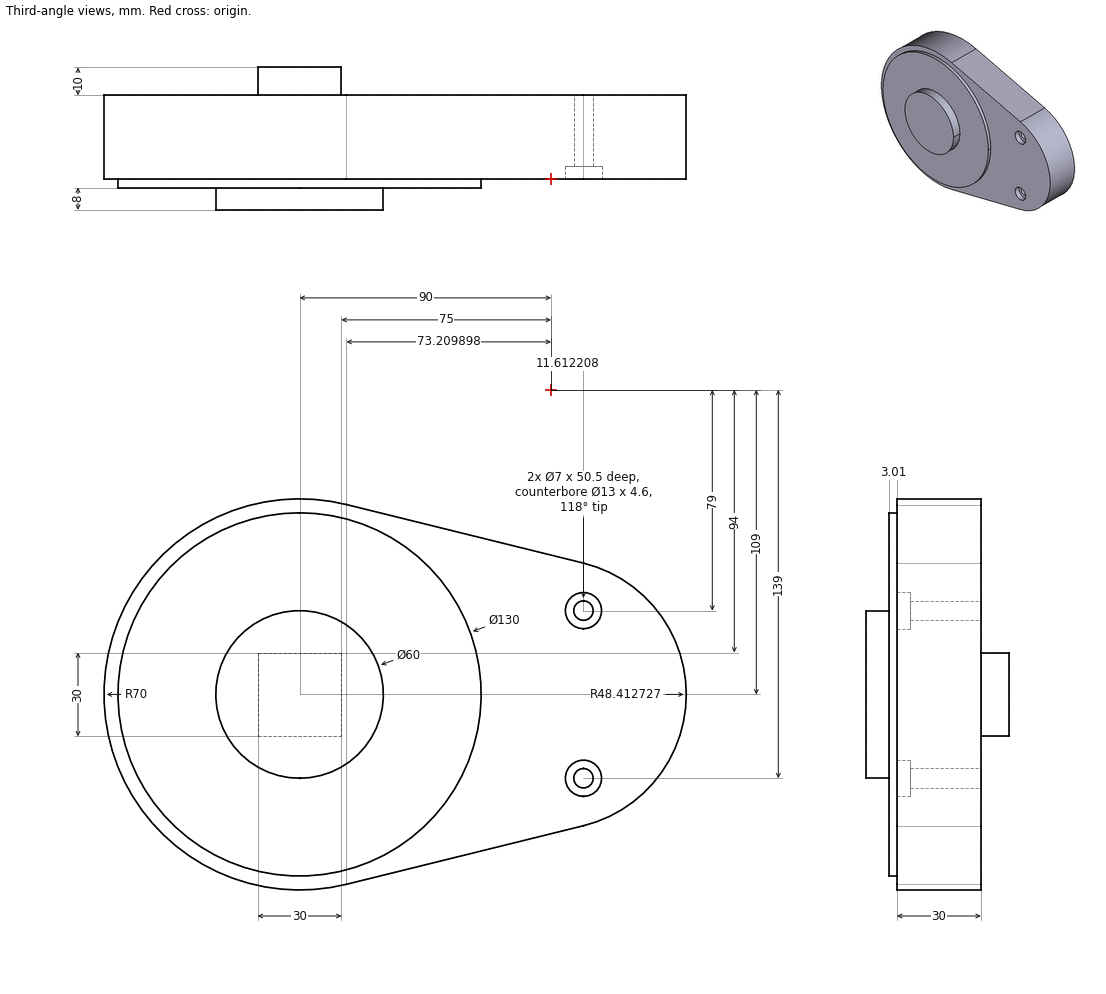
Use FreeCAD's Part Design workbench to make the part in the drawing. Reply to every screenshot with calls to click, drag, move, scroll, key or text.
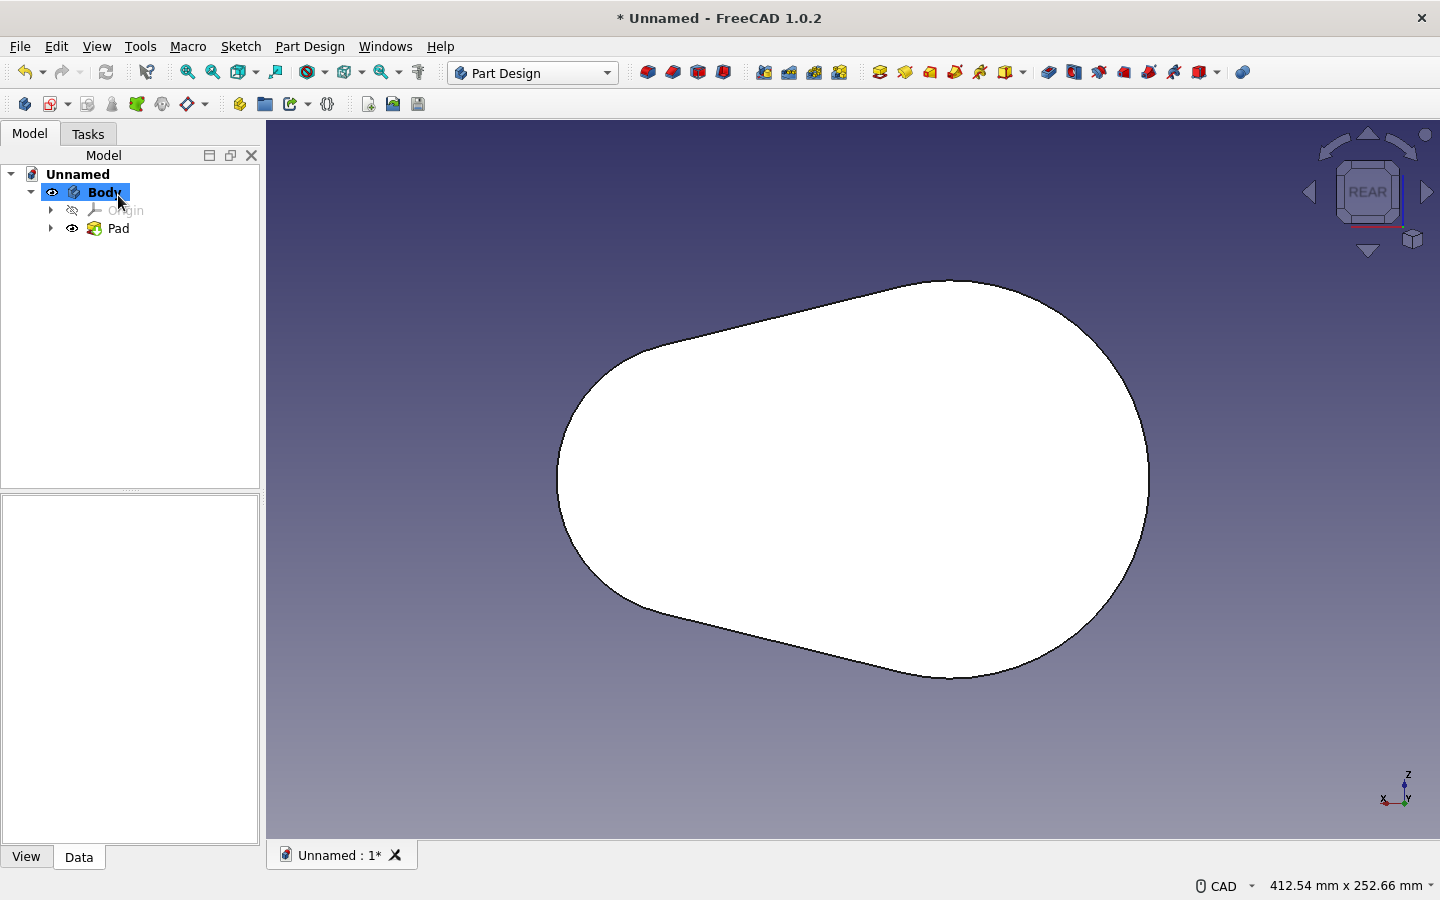
click(938, 478)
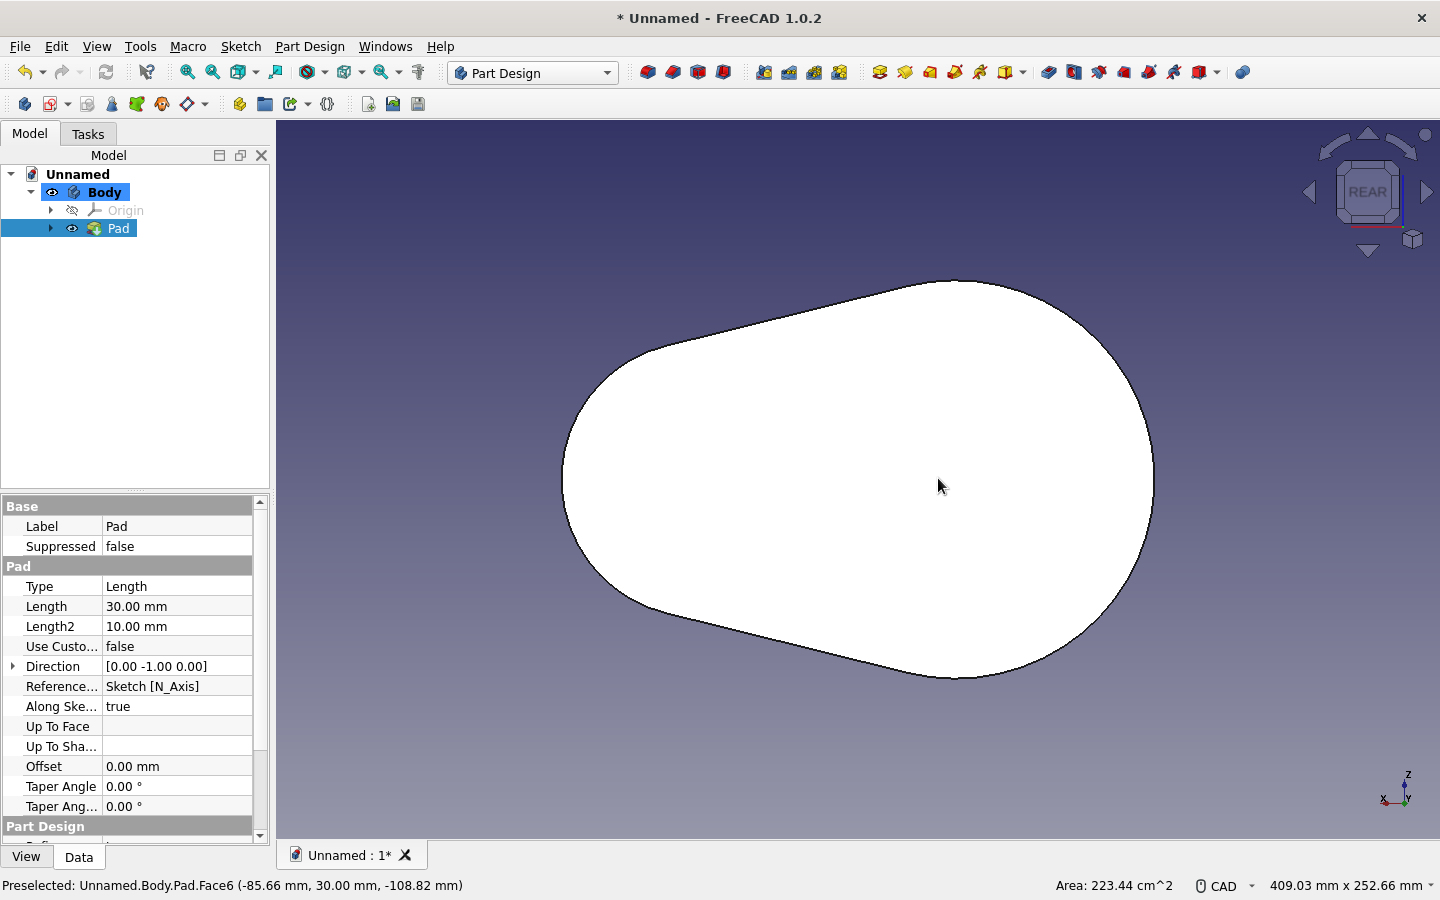
click(50, 104)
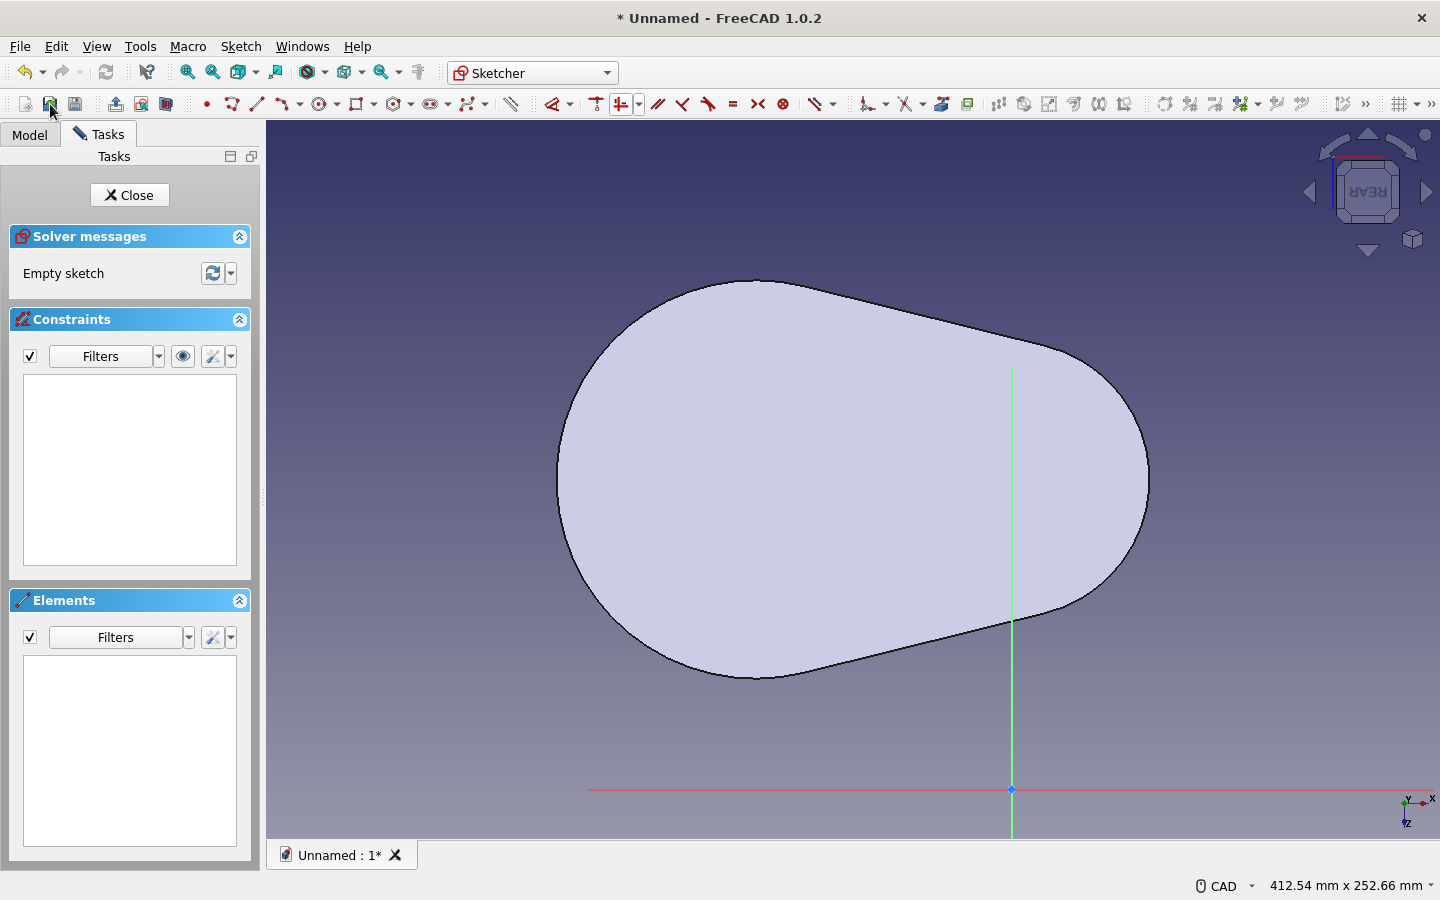
scroll(750, 480, up, 9)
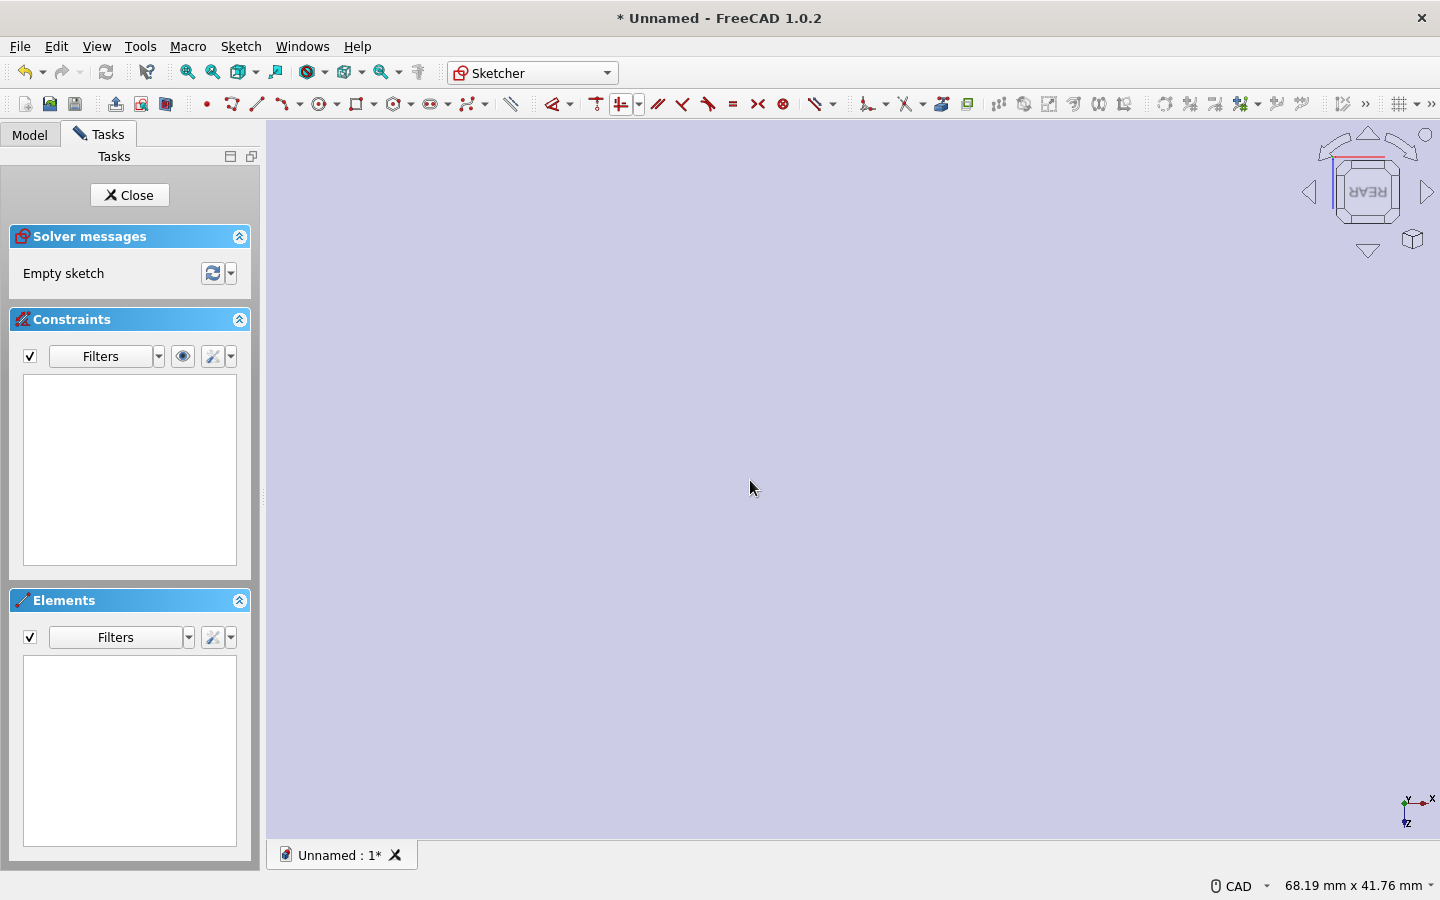
key(g)
key(r)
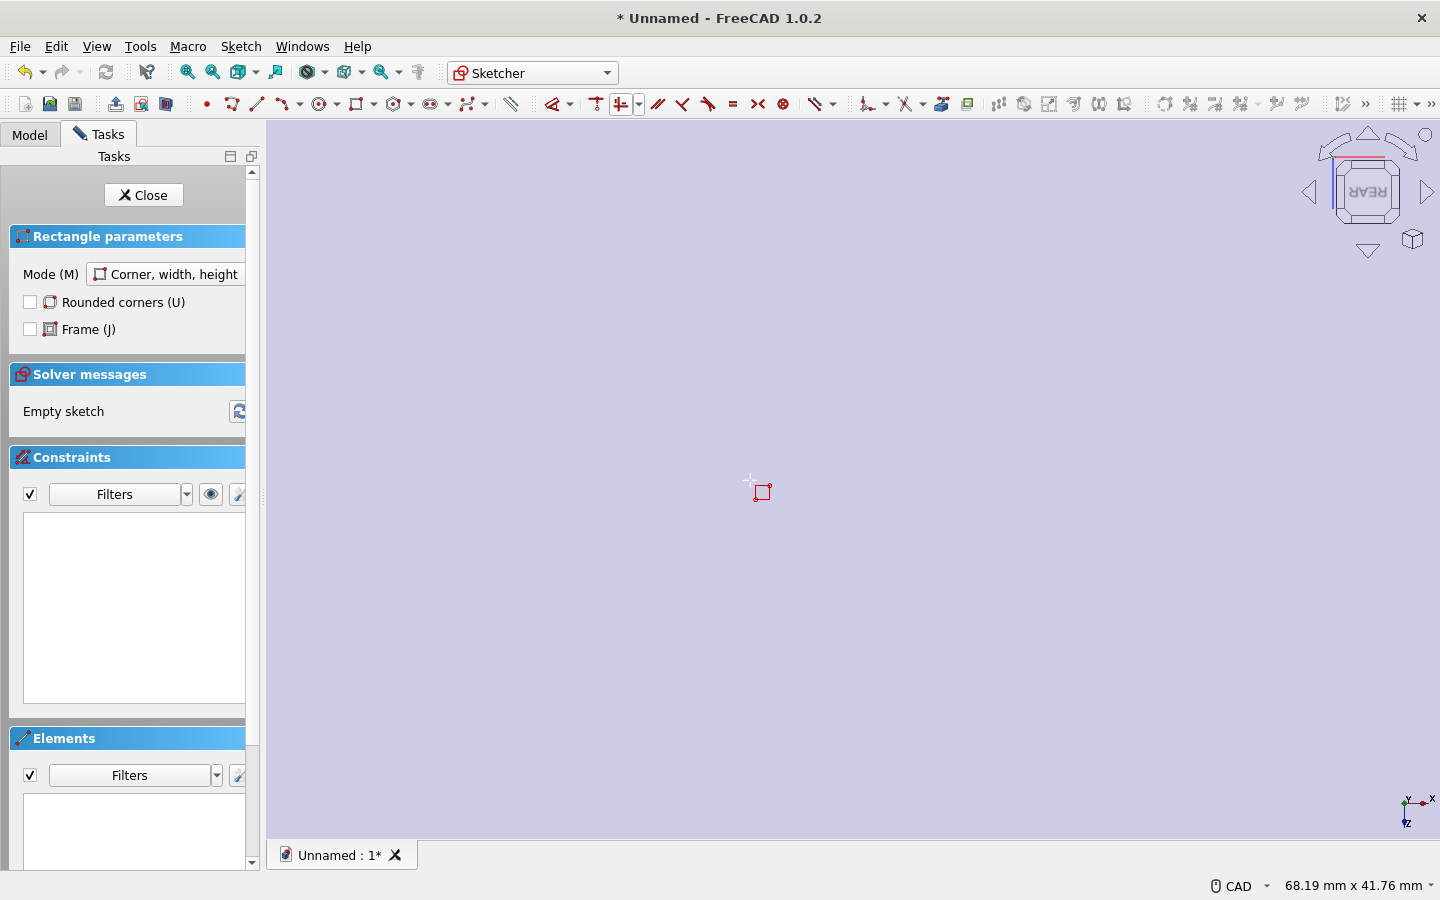
click(524, 216)
click(1040, 733)
key(Escape)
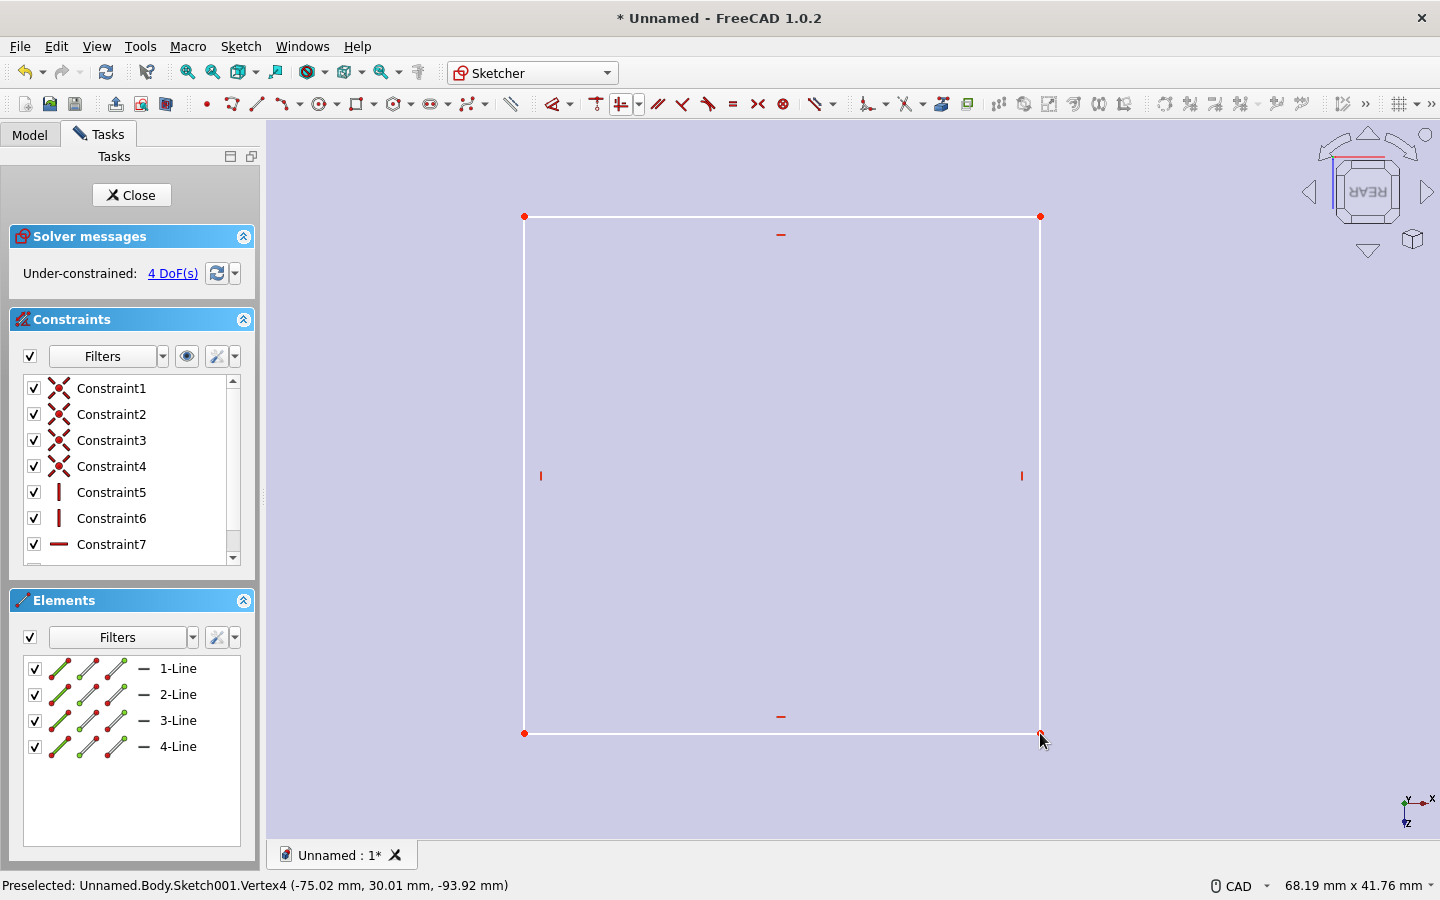
key(d)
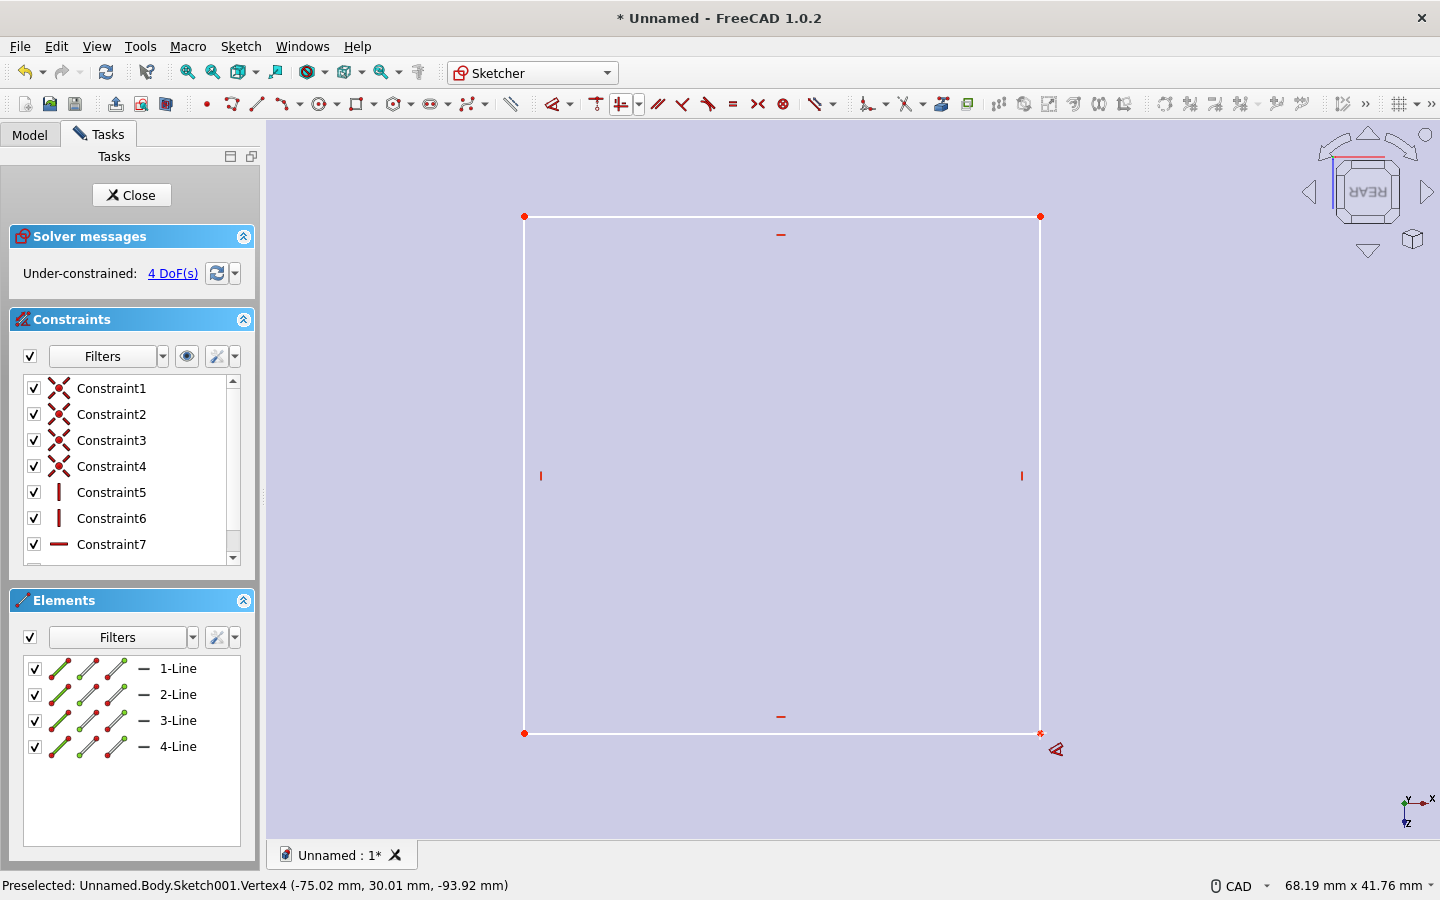
click(524, 372)
click(490, 475)